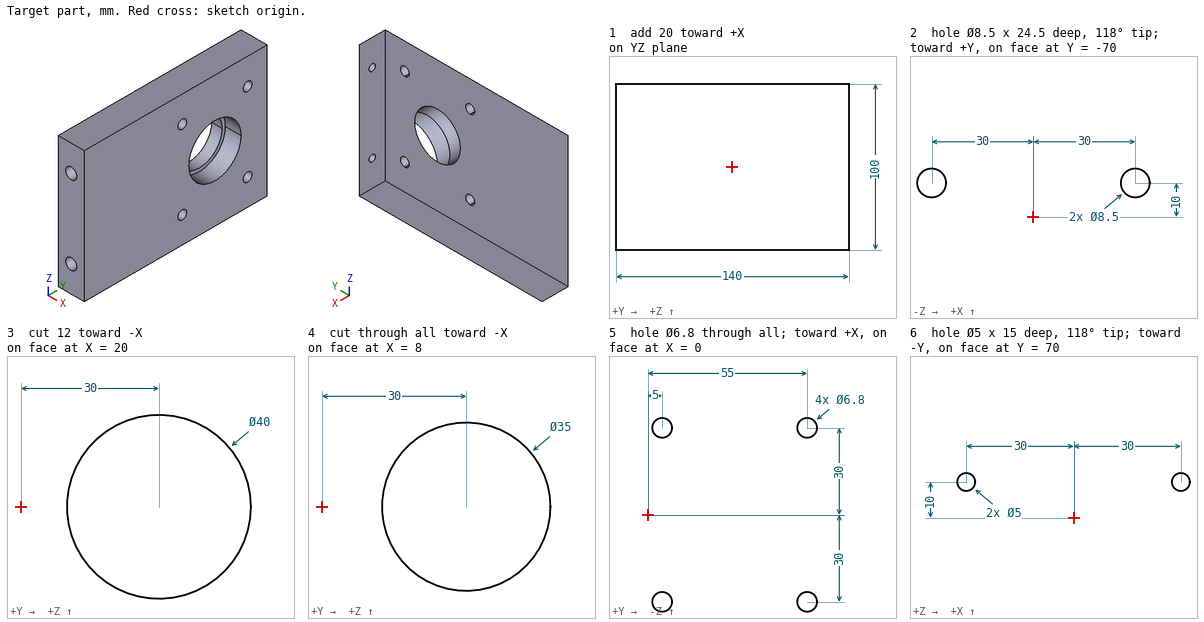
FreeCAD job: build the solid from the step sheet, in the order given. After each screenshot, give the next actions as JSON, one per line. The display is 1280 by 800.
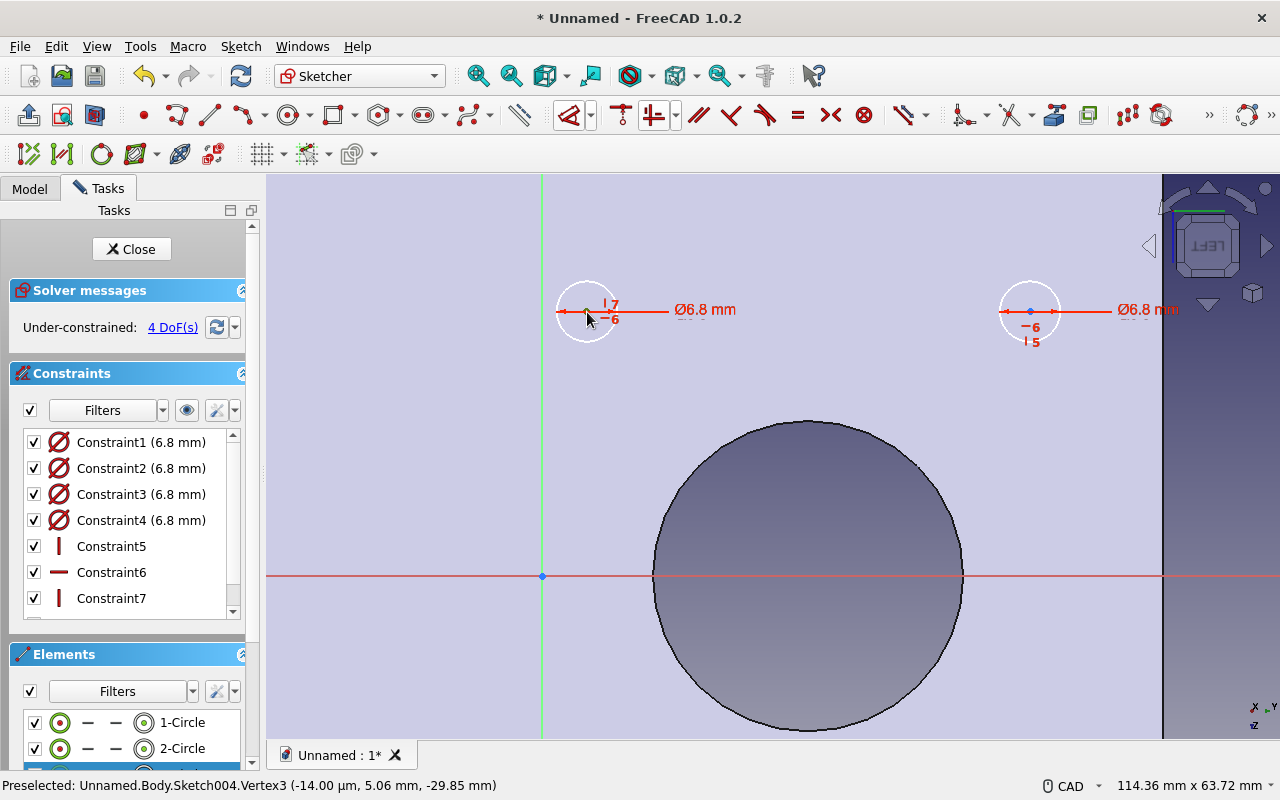
{"action": "key", "text": "l"}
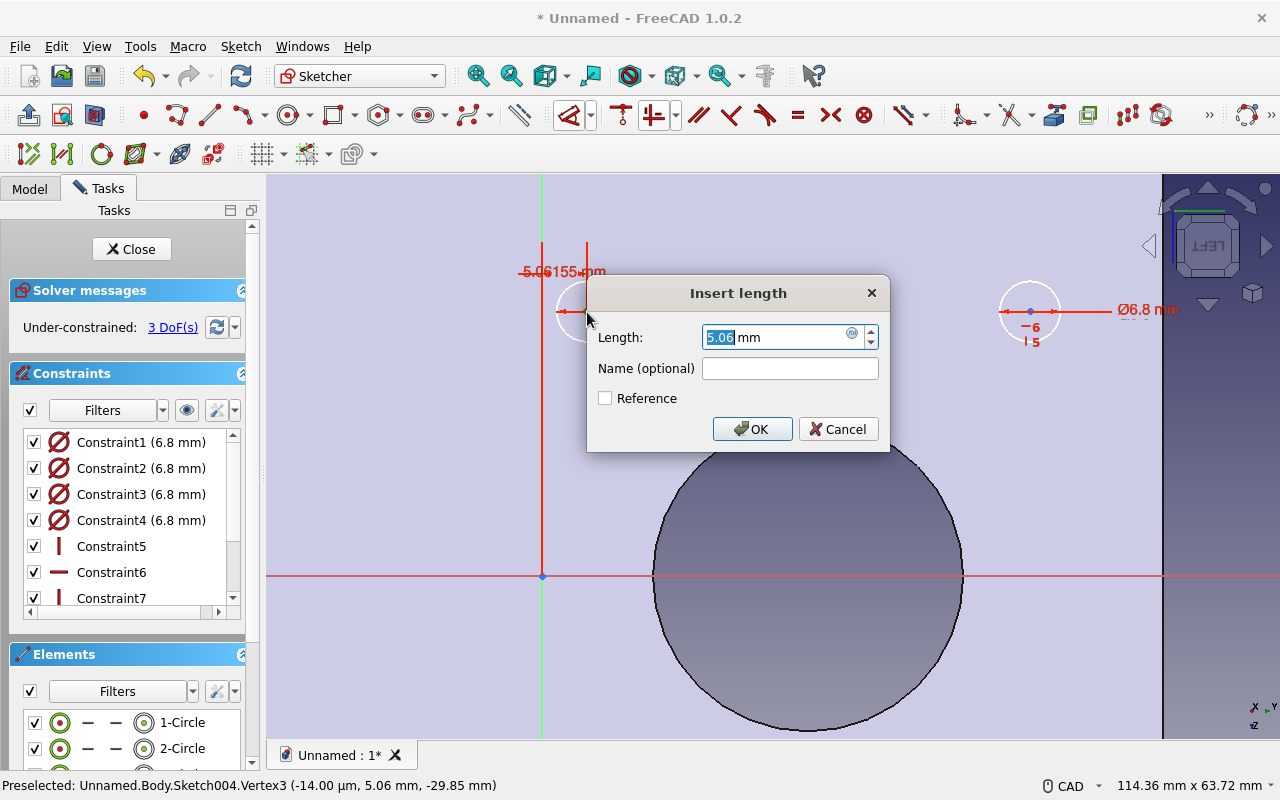
{"action": "type", "text": "5"}
{"action": "key", "text": "Return"}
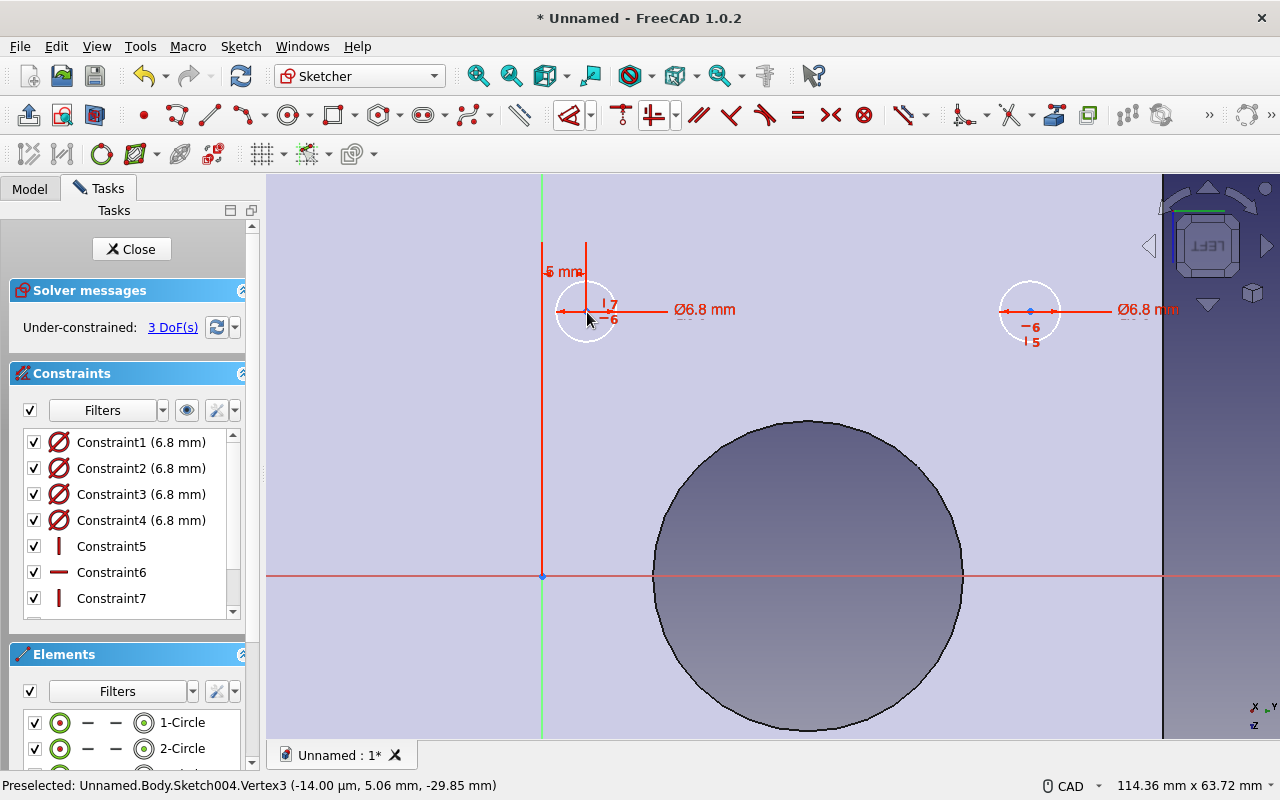
{"action": "left_click", "coordinate": [1030, 312]}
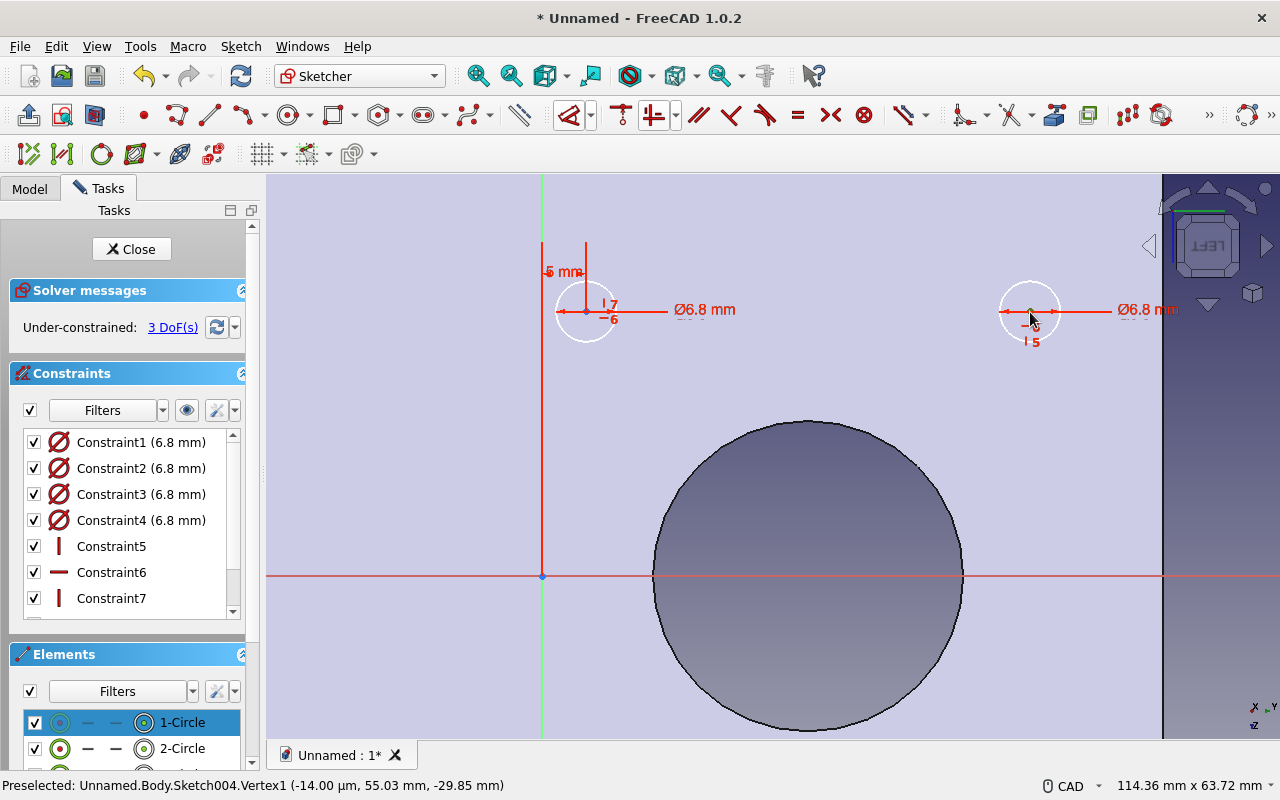
{"action": "left_click", "coordinate": [590, 116]}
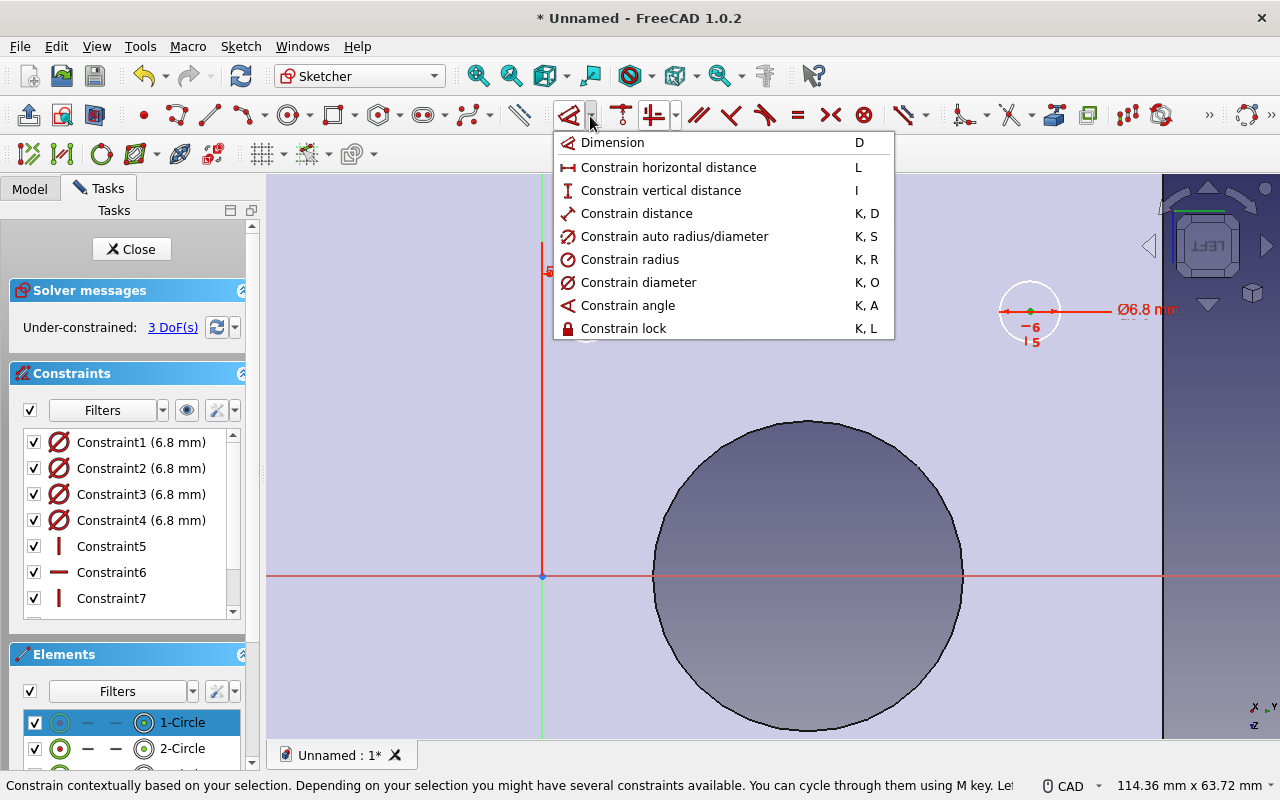
{"action": "left_click", "coordinate": [724, 168]}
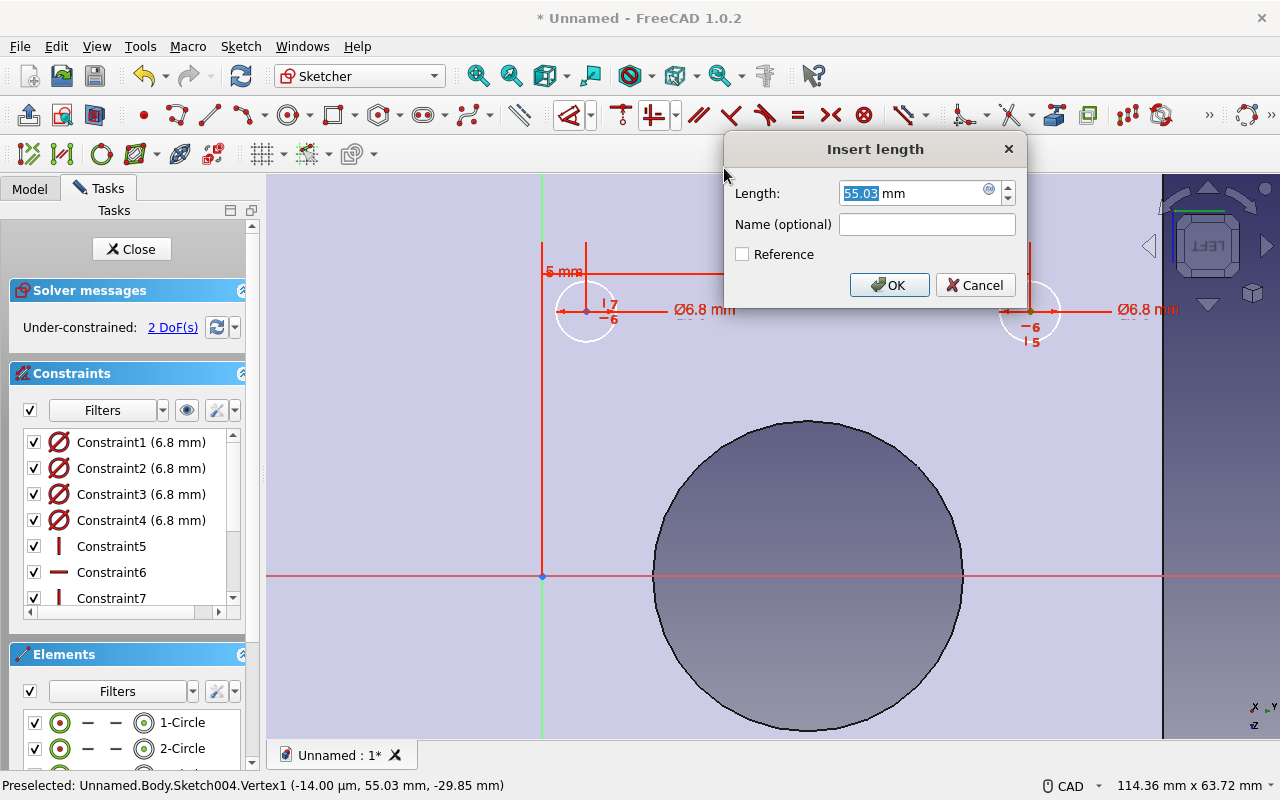
{"action": "type", "text": "55"}
{"action": "key", "text": "Return"}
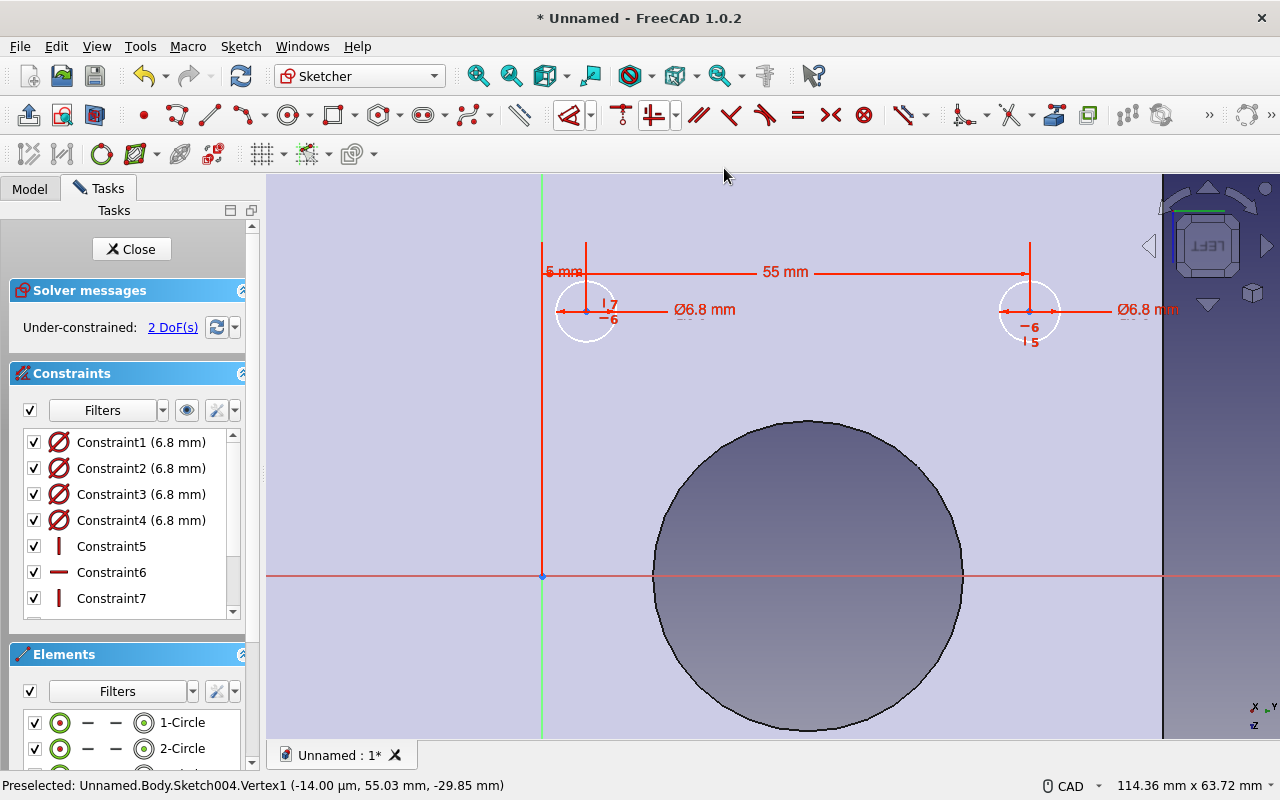
{"action": "left_click", "coordinate": [1030, 312]}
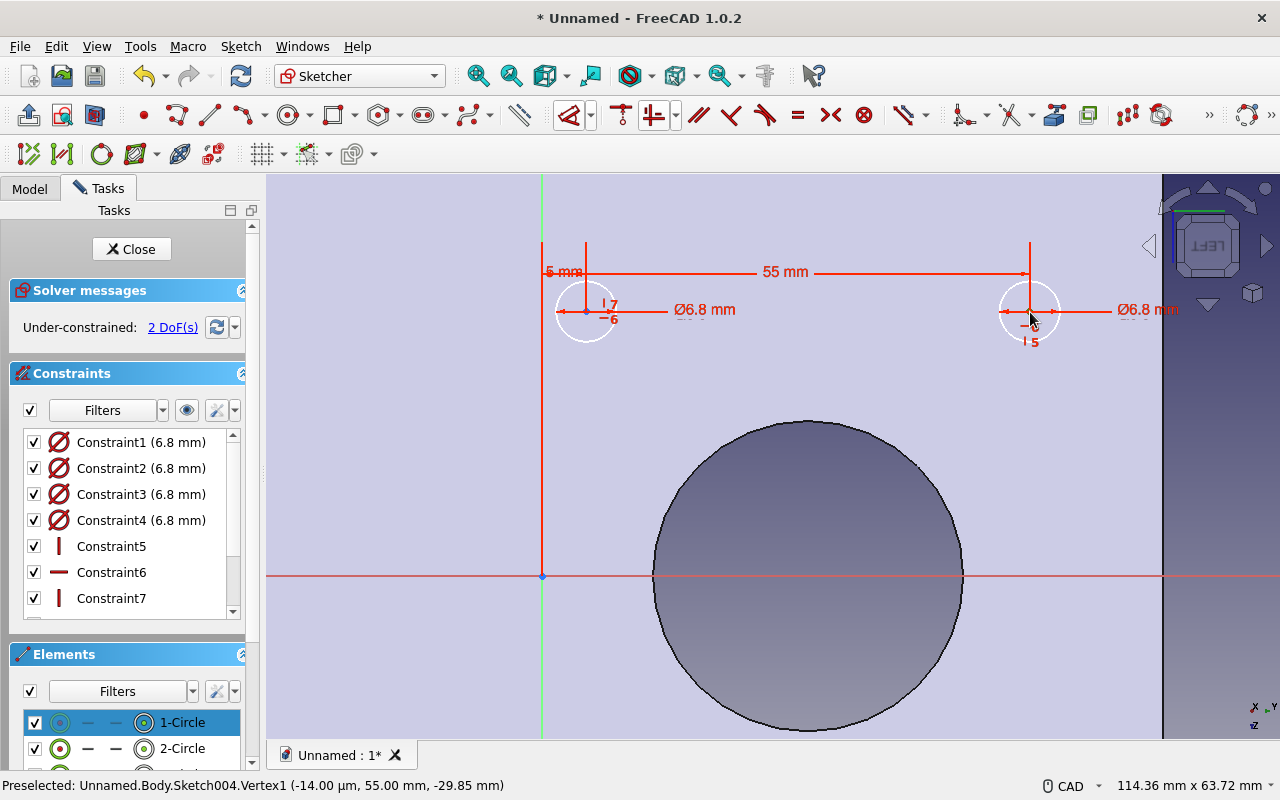
{"action": "key", "text": "i"}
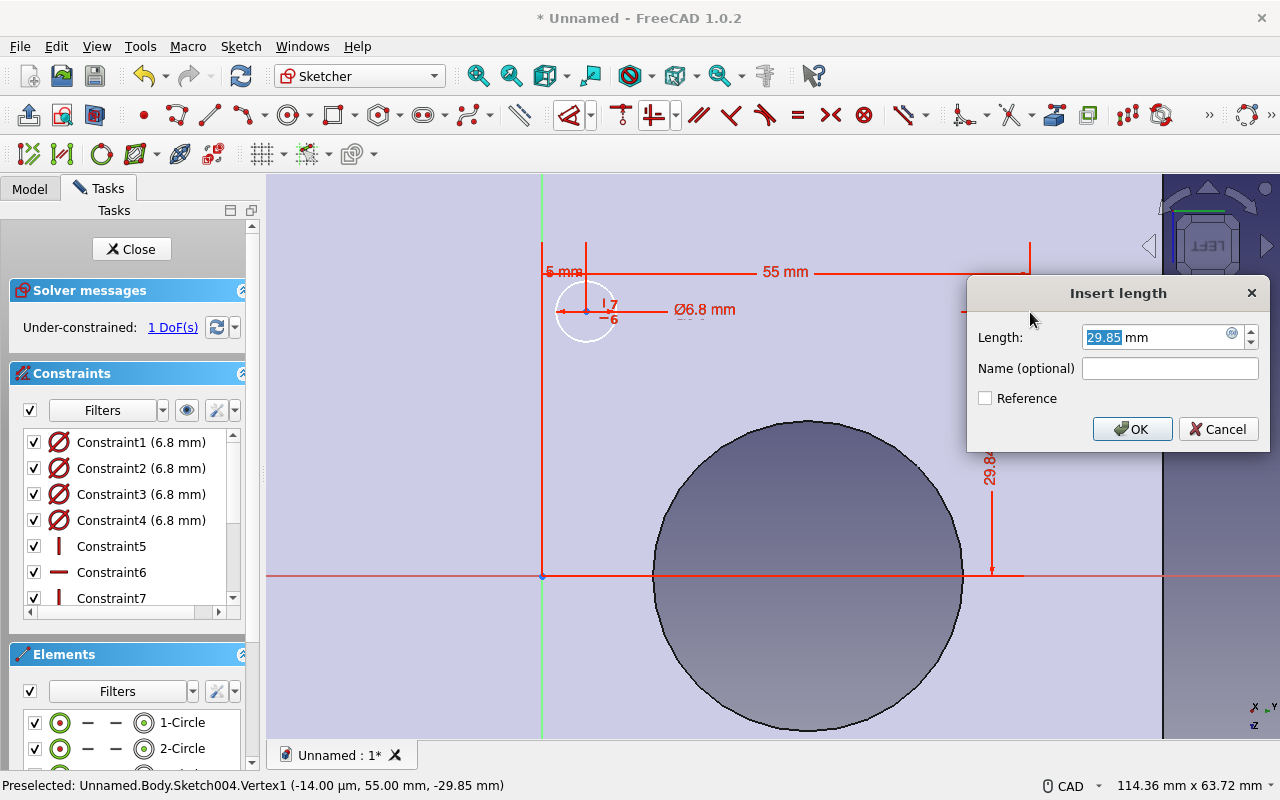
{"action": "type", "text": "30"}
{"action": "key", "text": "Return"}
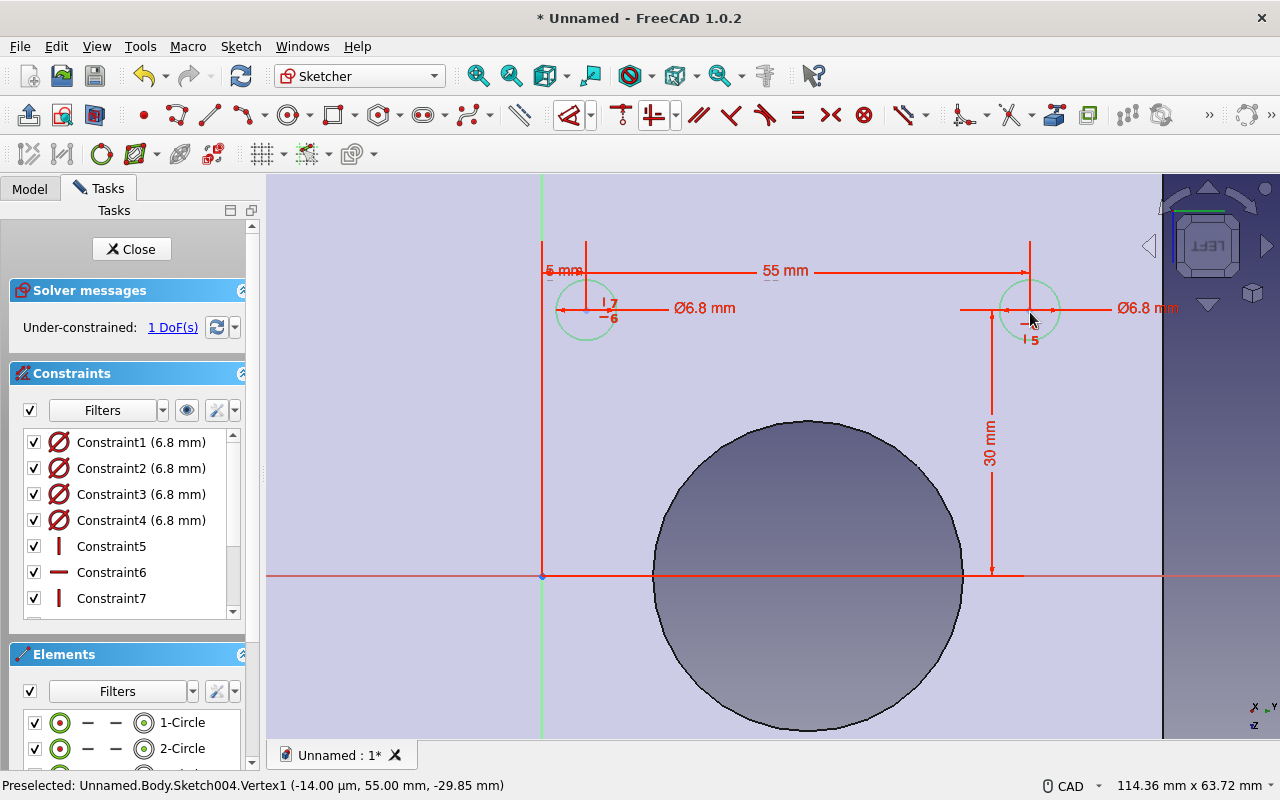
{"action": "scroll", "coordinate": [587, 311], "scroll_direction": "down", "scroll_amount": 3}